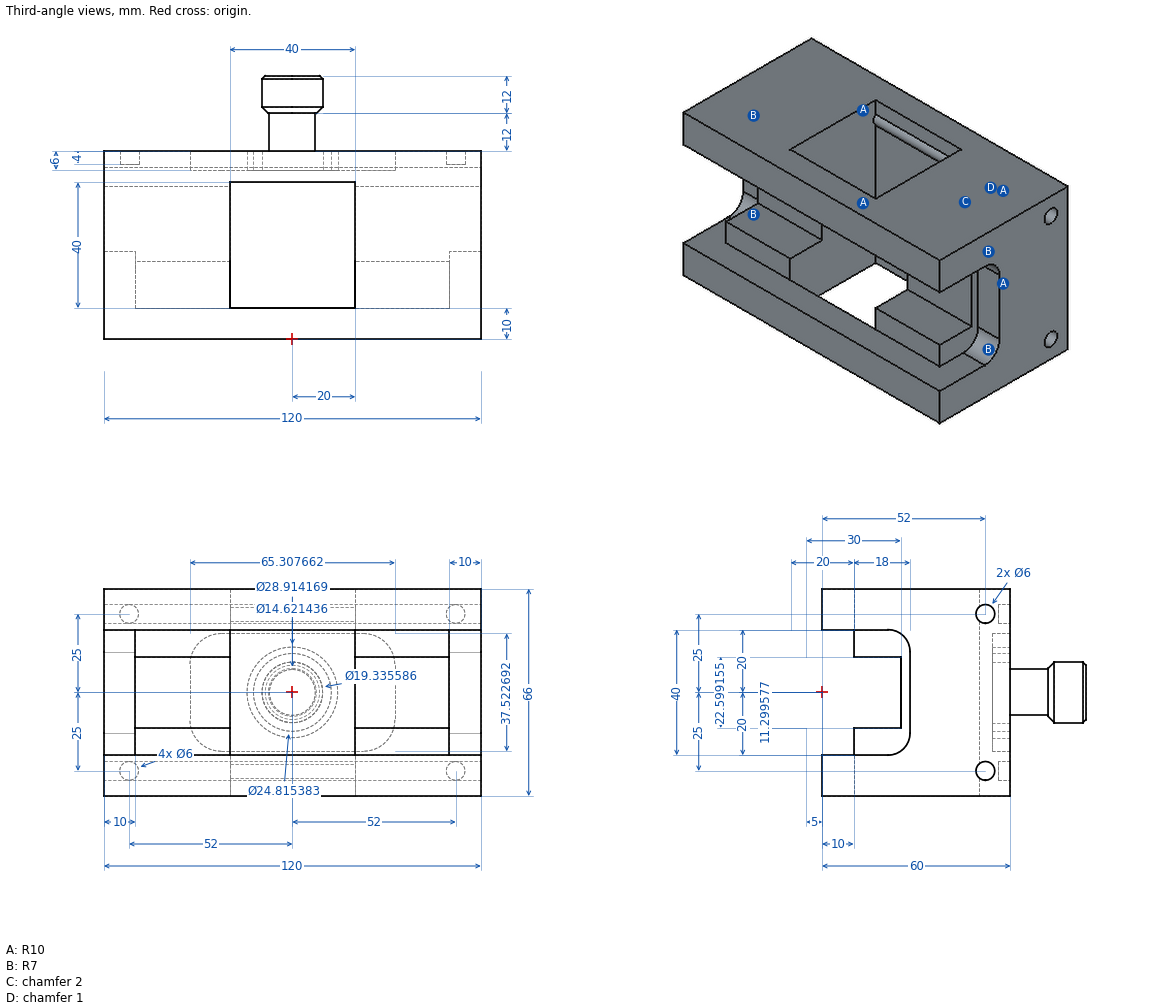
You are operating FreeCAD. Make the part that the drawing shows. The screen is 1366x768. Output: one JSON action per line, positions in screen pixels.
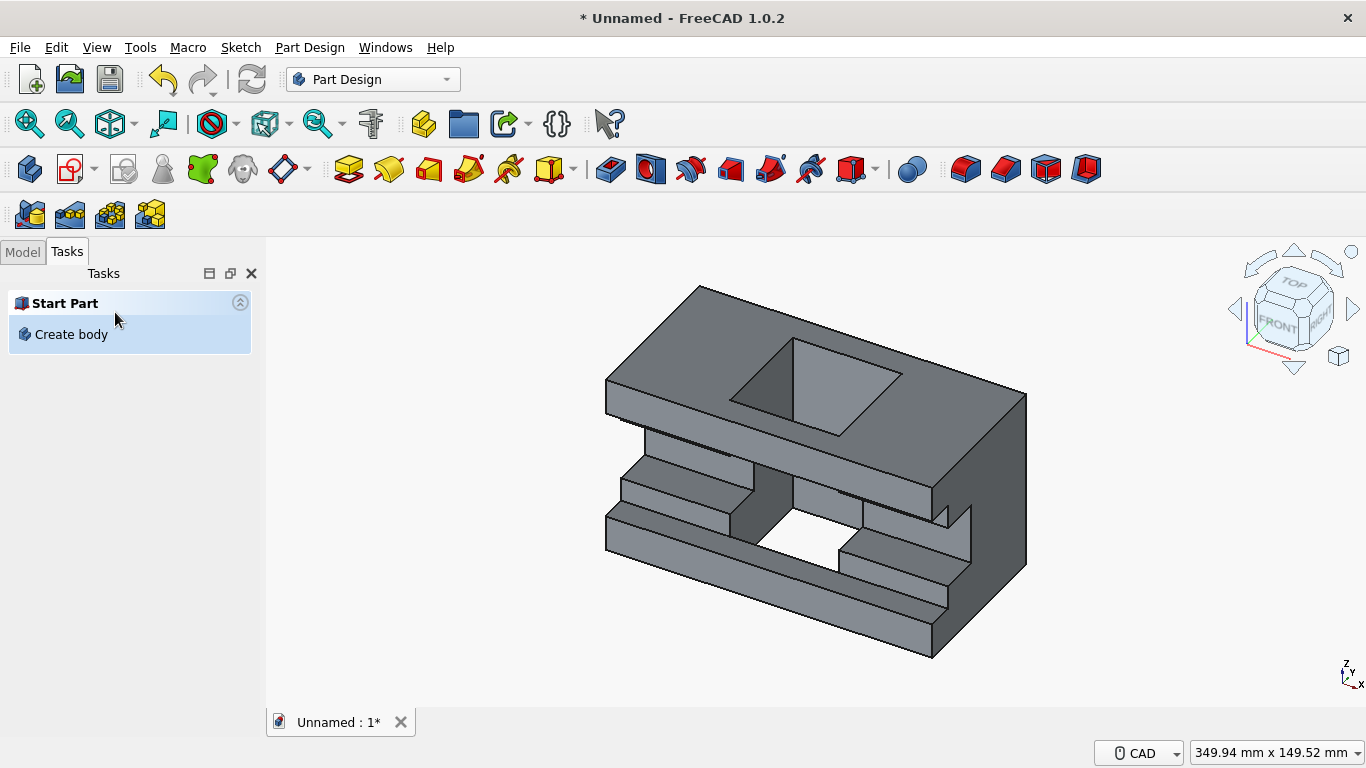
{"action": "left_click", "coordinate": [993, 463]}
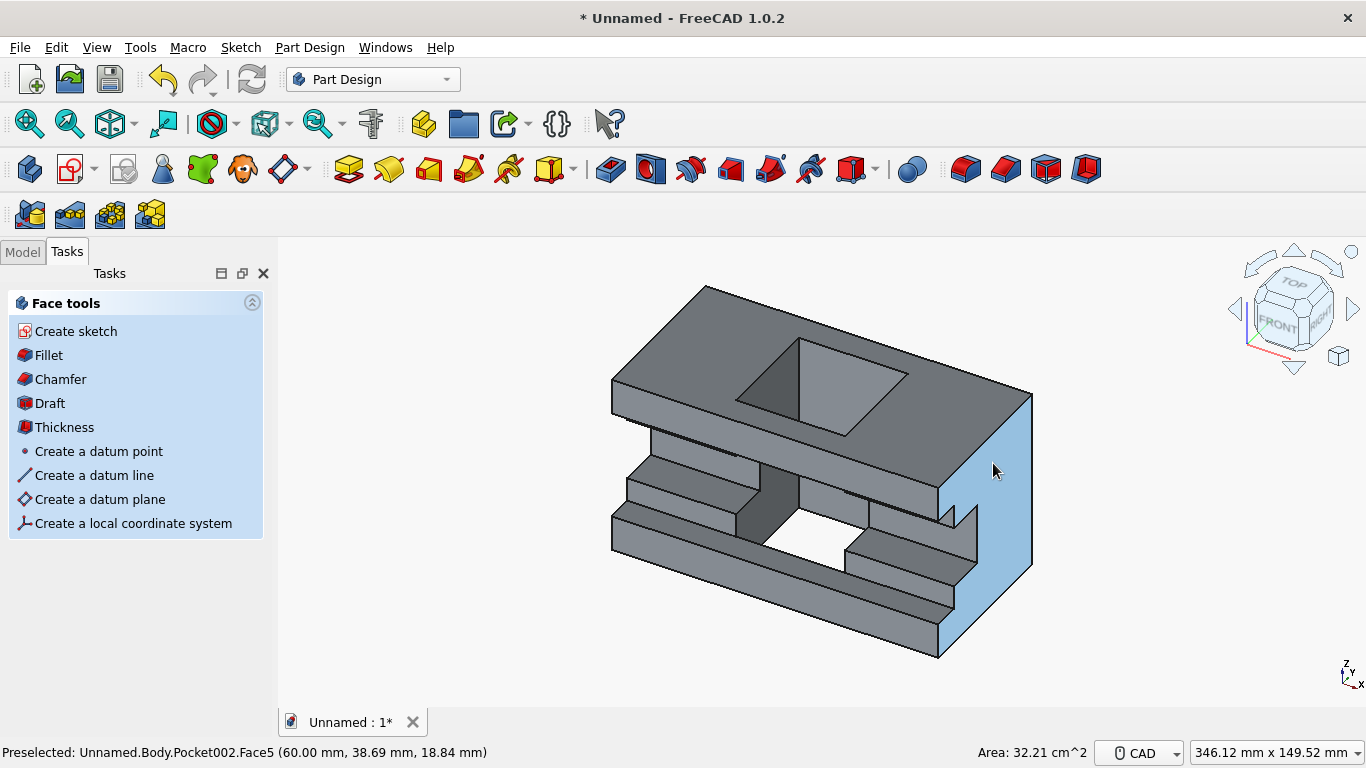
{"action": "left_click", "coordinate": [70, 170]}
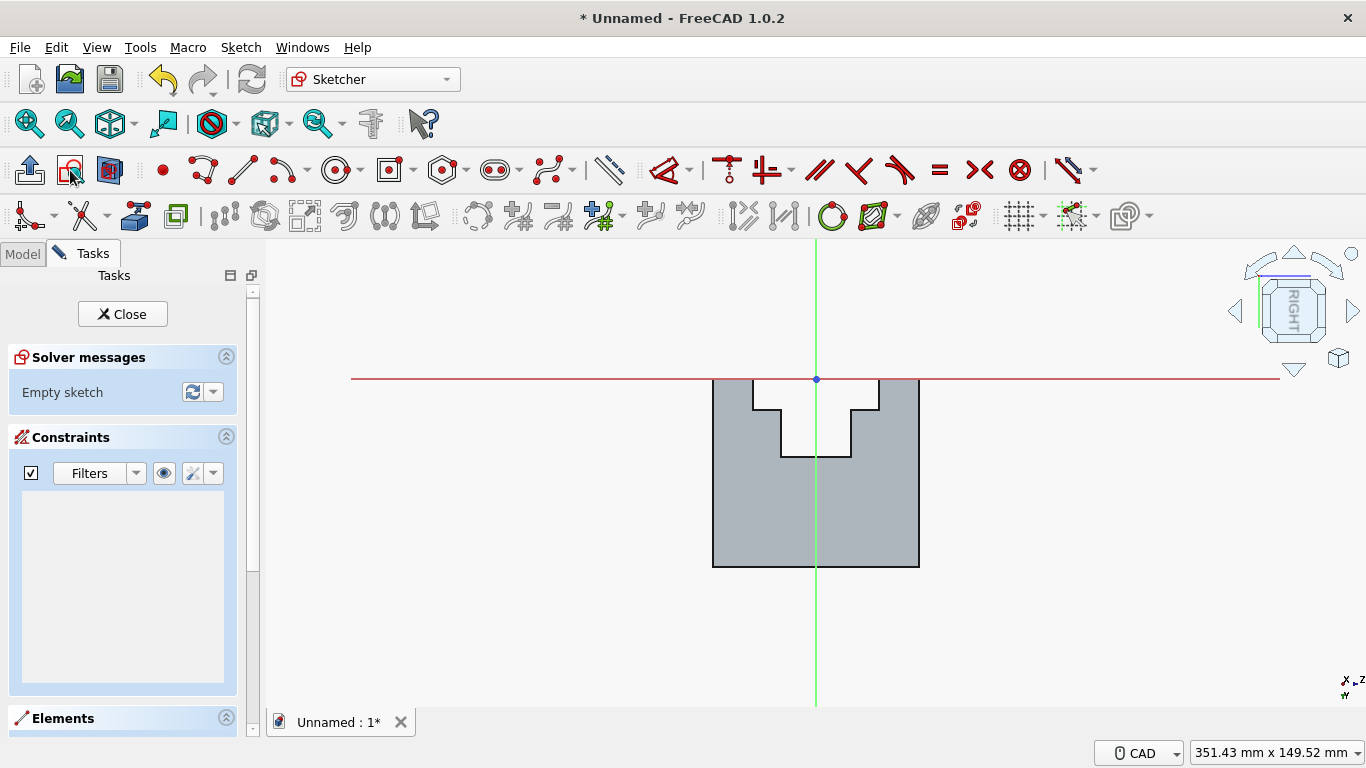
{"action": "scroll", "coordinate": [899, 456], "scroll_direction": "up", "scroll_amount": 3}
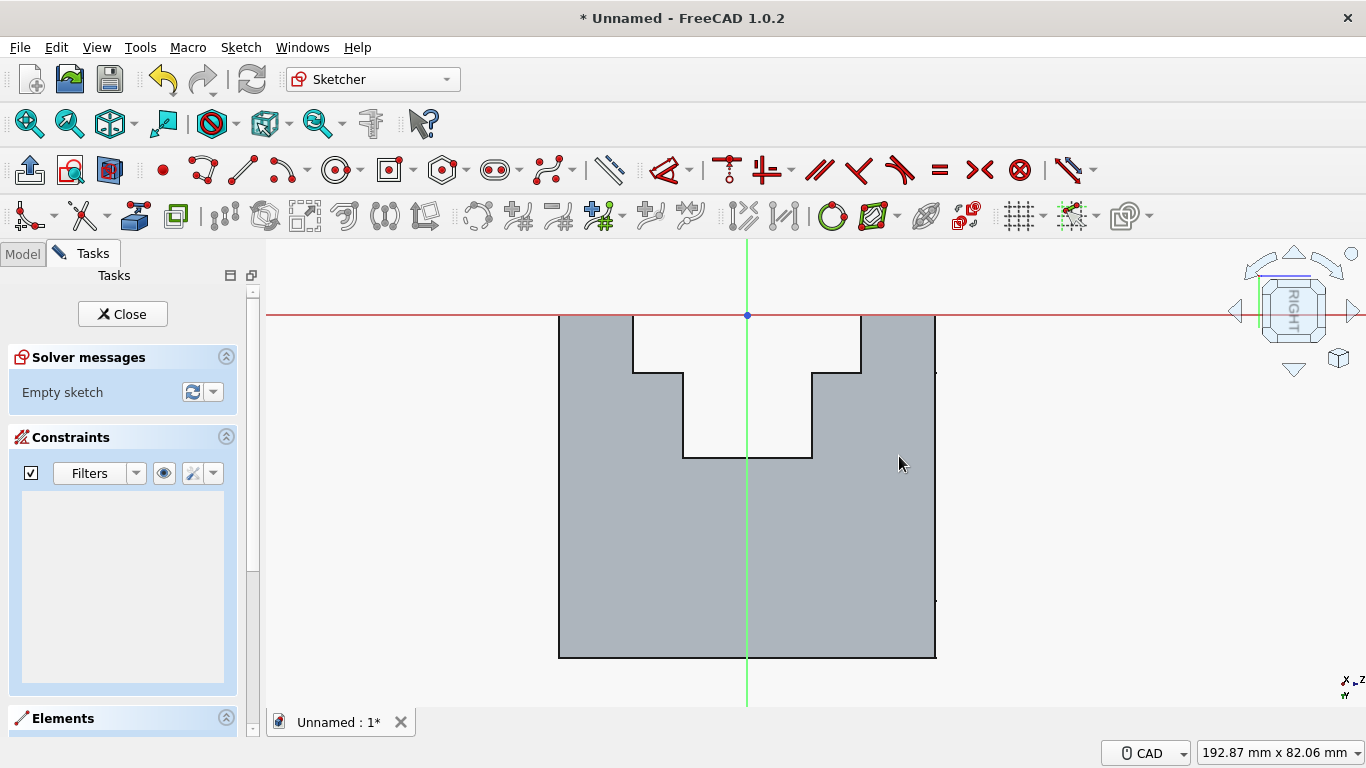
{"action": "left_click", "coordinate": [336, 170]}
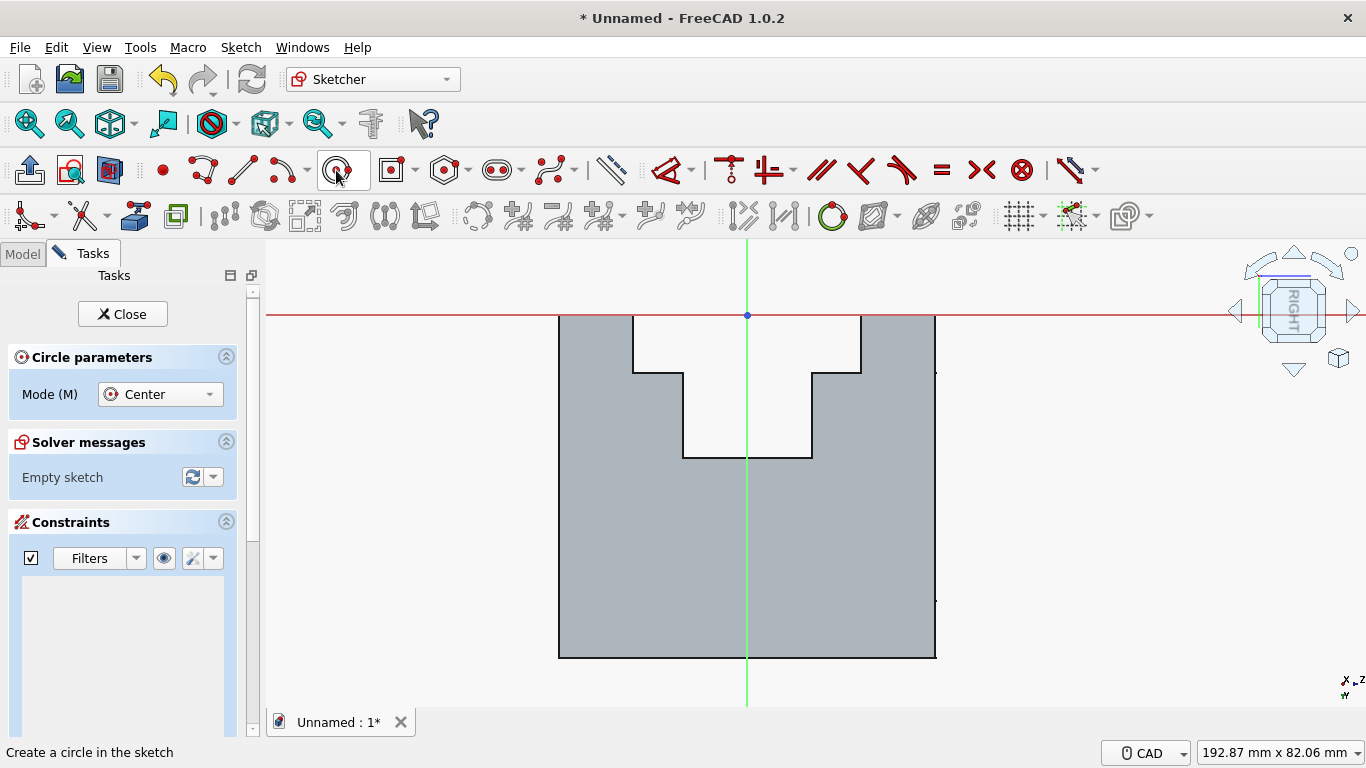
{"action": "scroll", "coordinate": [890, 612], "scroll_direction": "up", "scroll_amount": 2}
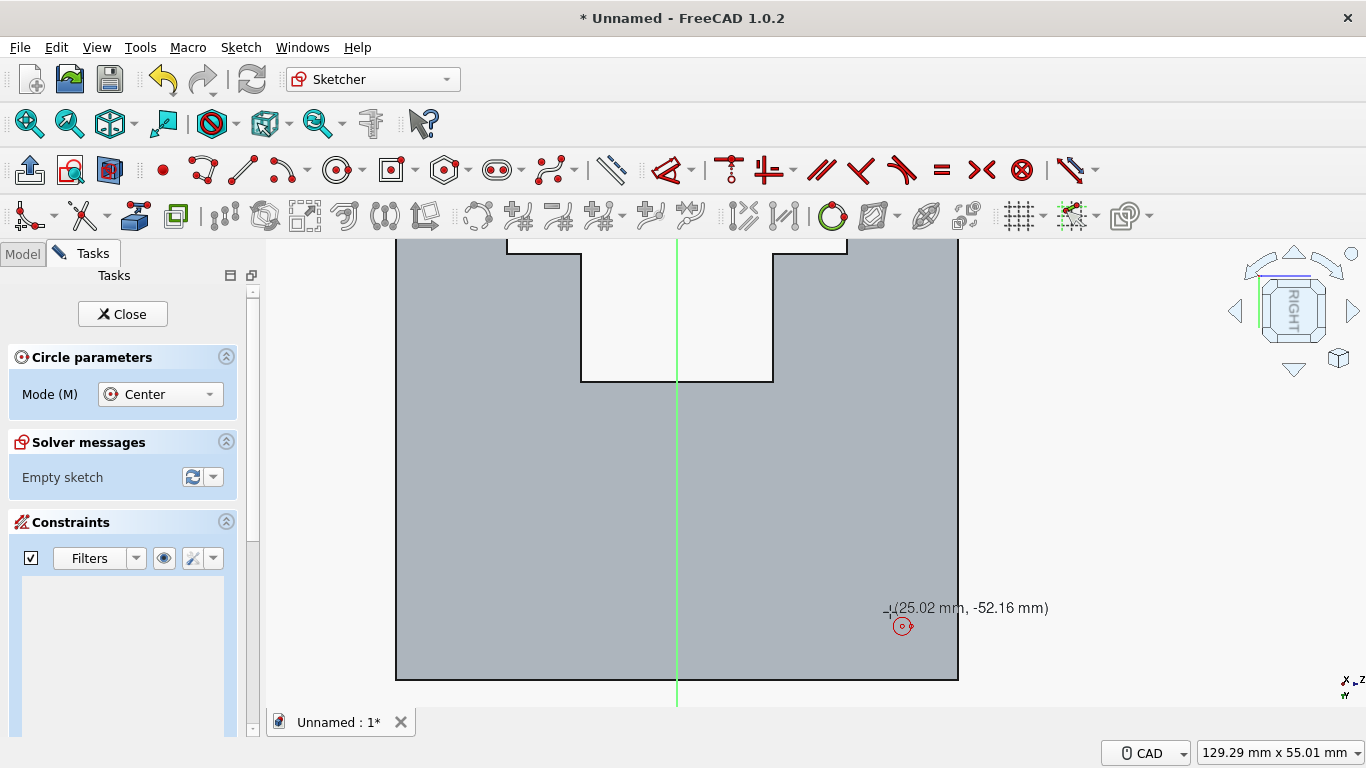
{"action": "left_click", "coordinate": [890, 612]}
{"action": "mouse_move", "coordinate": [908, 594]}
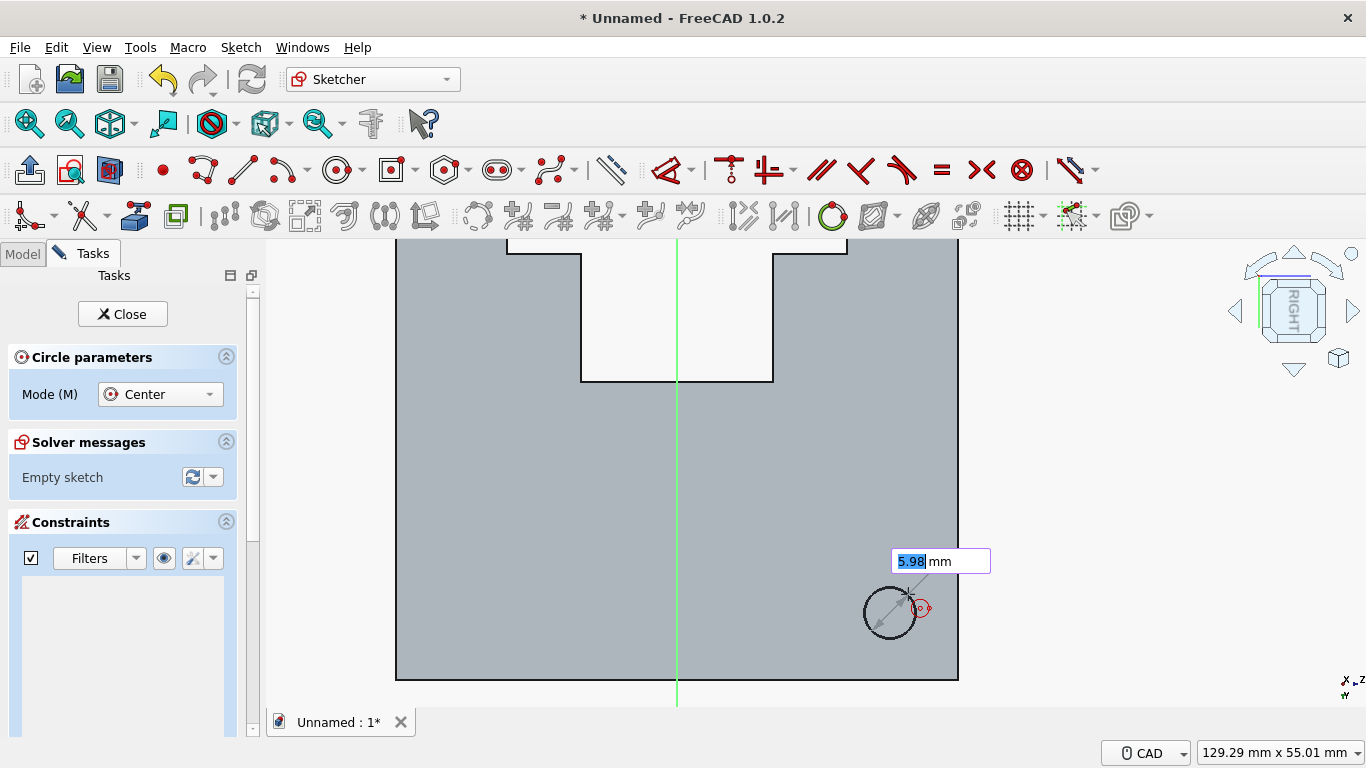
{"action": "type", "text": "6"}
{"action": "key", "text": "Return"}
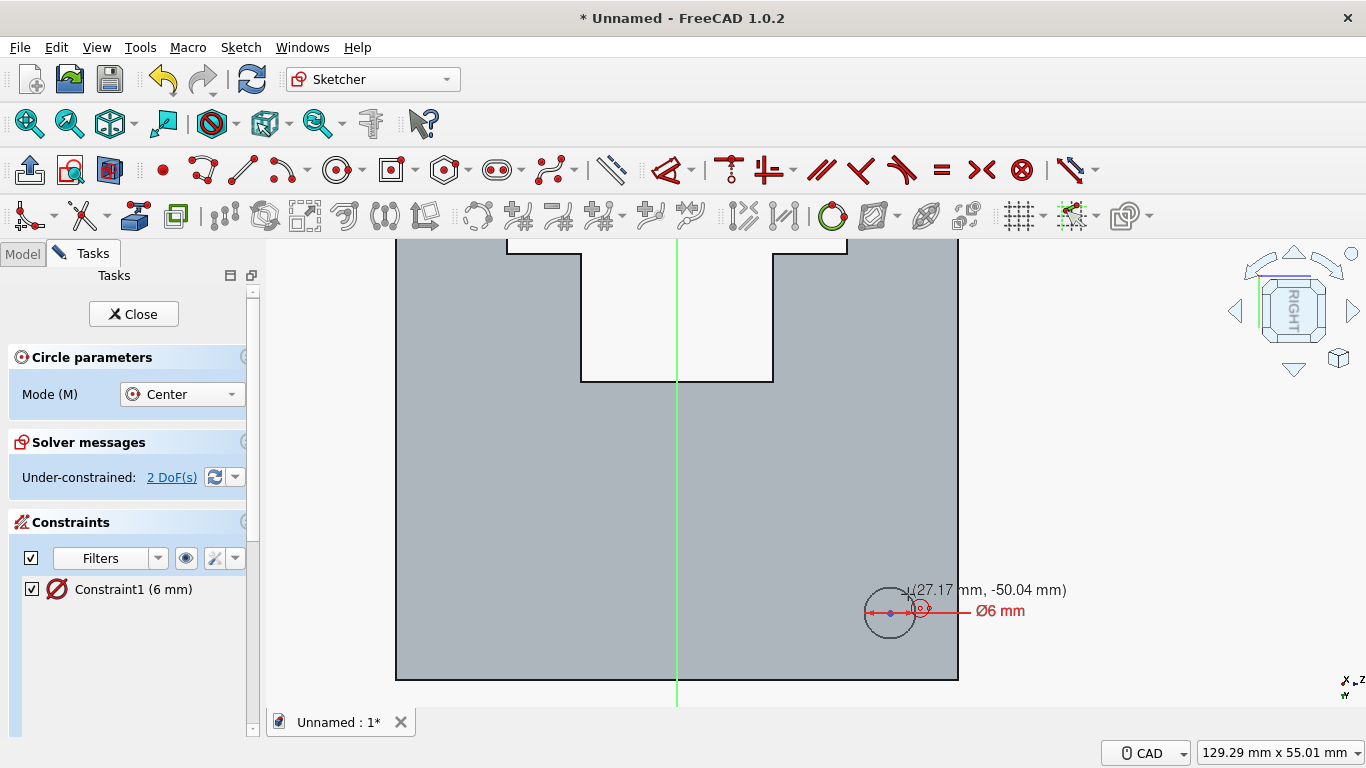
{"action": "left_click", "coordinate": [464, 612]}
{"action": "mouse_move", "coordinate": [482, 594]}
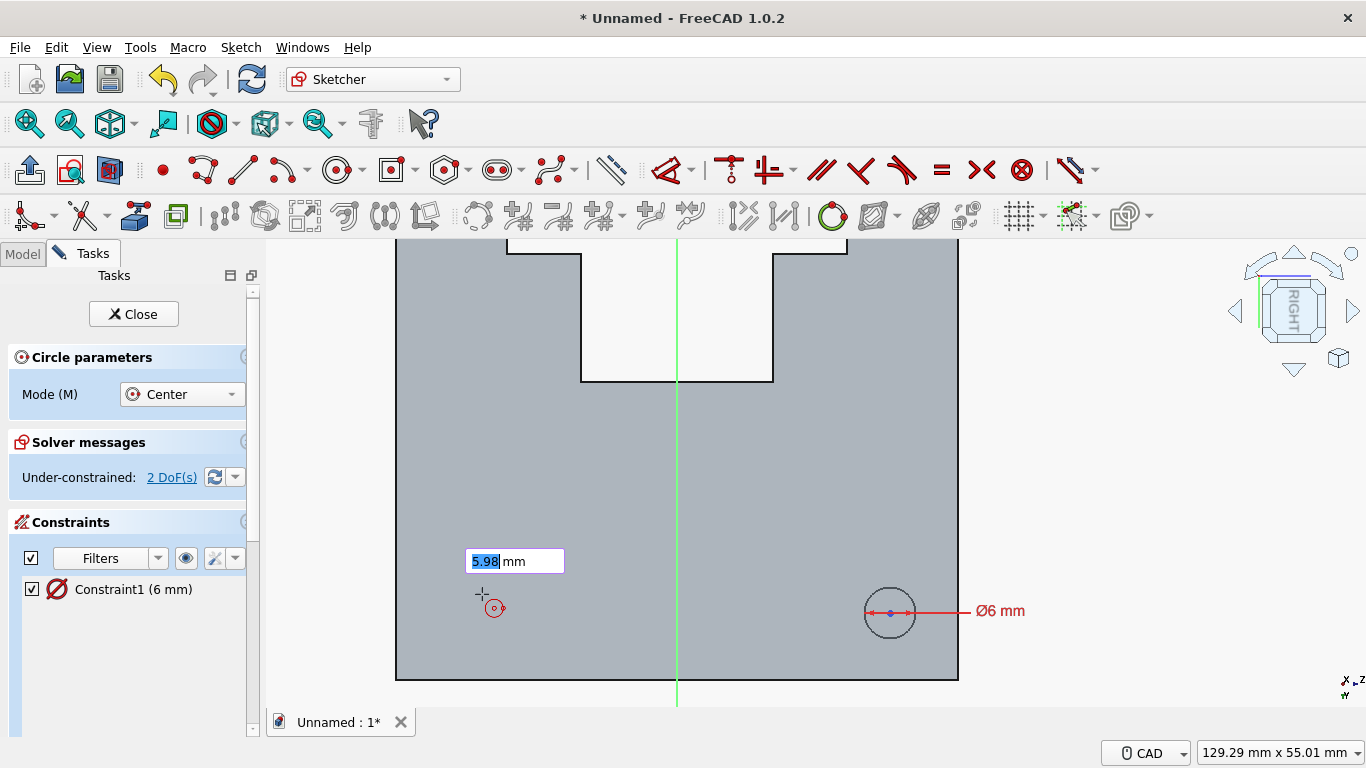
{"action": "type", "text": "6"}
{"action": "key", "text": "Return"}
{"action": "key", "text": "Escape"}